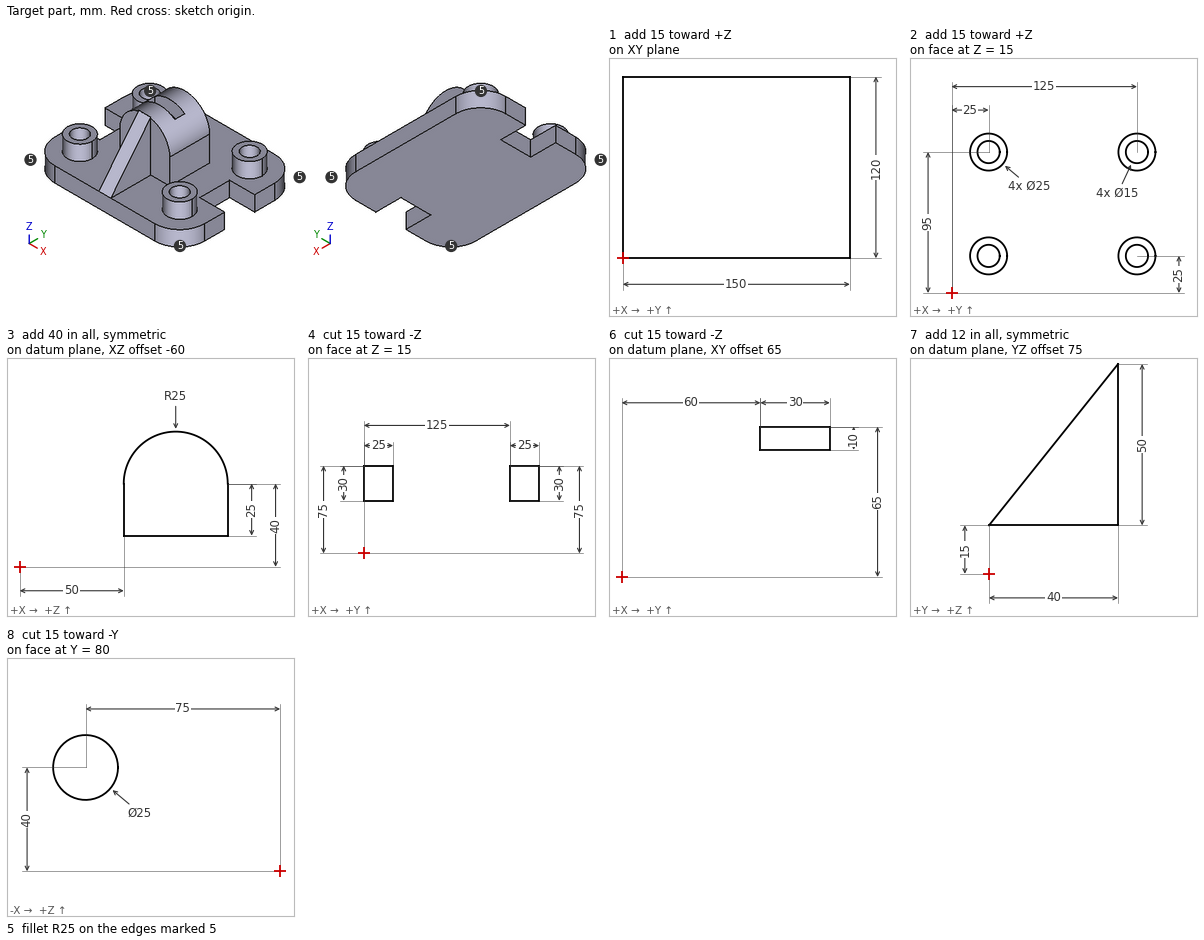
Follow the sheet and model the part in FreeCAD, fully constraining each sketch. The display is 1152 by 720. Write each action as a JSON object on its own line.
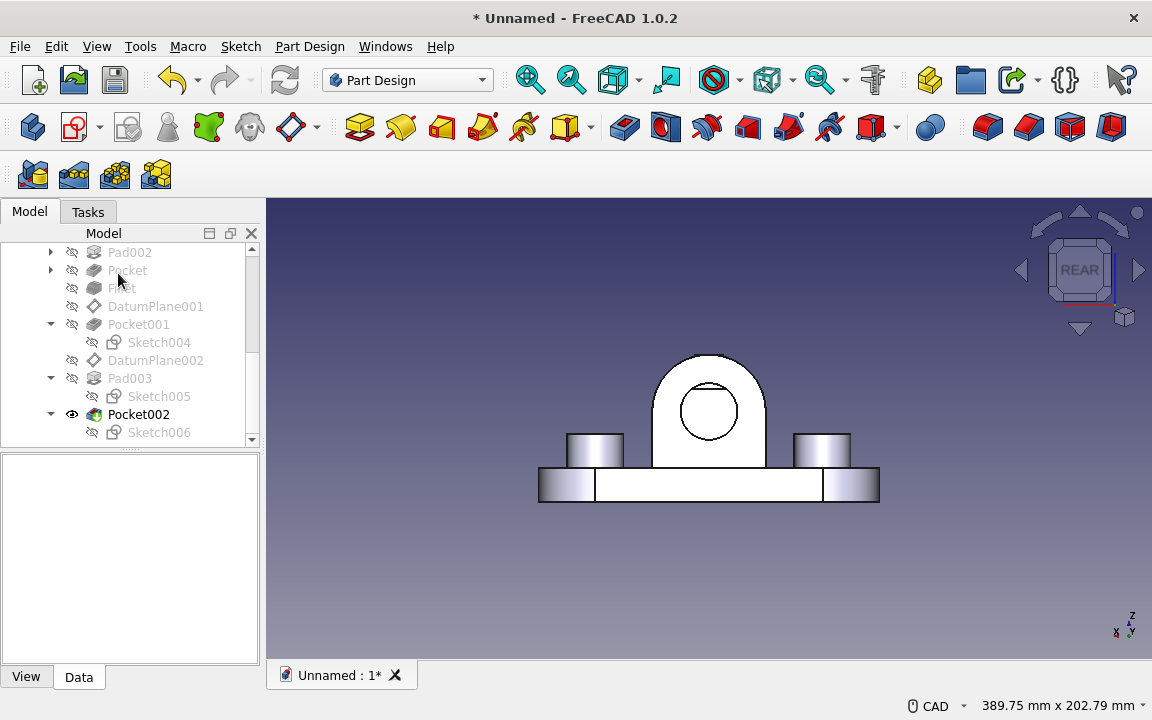
{"action": "key", "text": "0"}